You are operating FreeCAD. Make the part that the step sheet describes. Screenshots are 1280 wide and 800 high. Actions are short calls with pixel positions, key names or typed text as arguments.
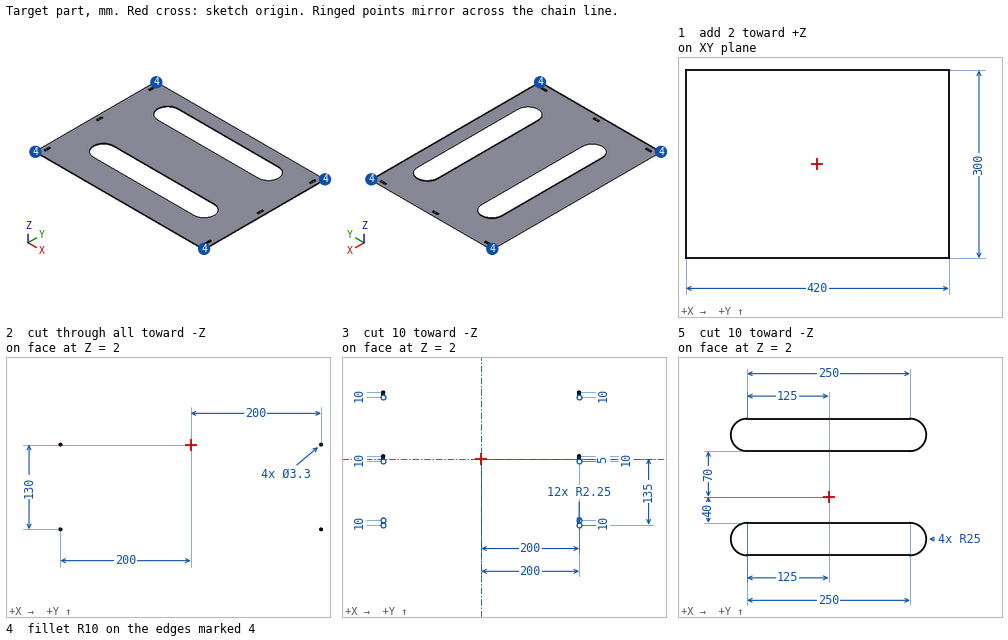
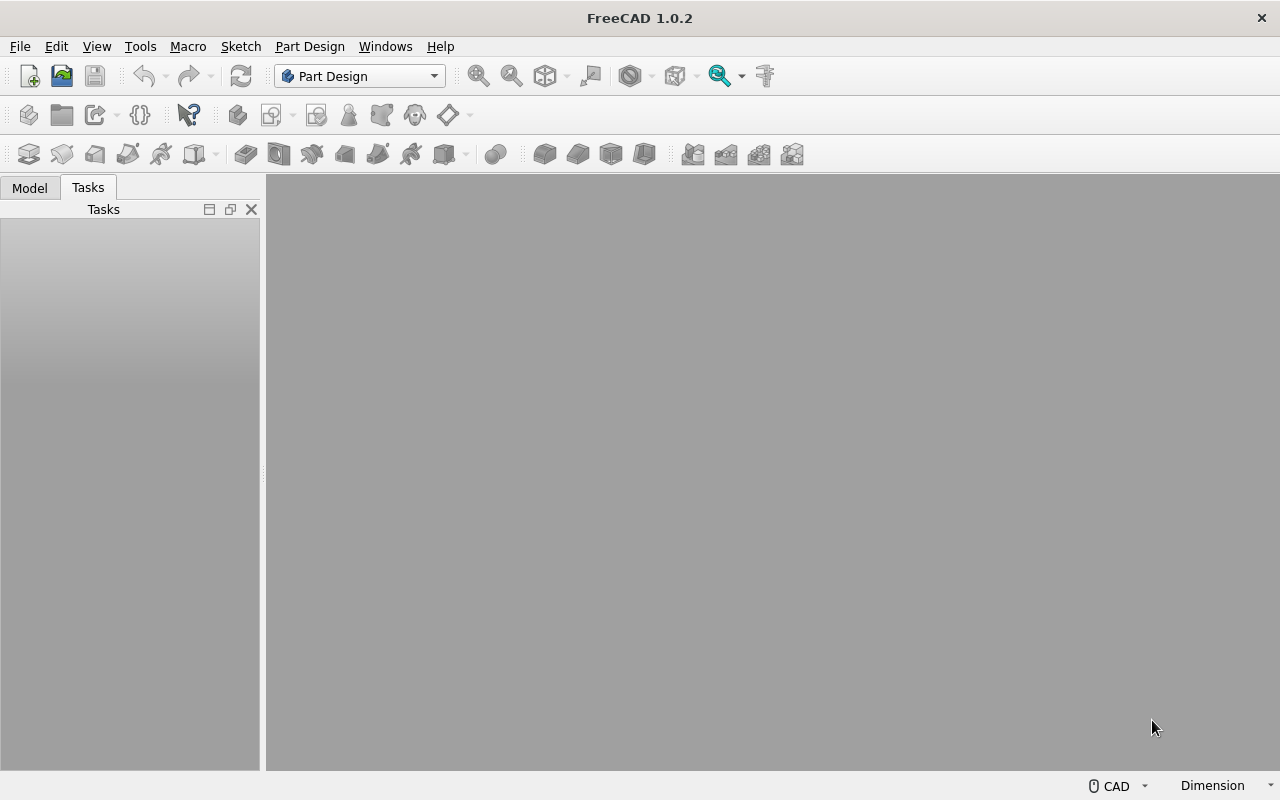
click(29, 76)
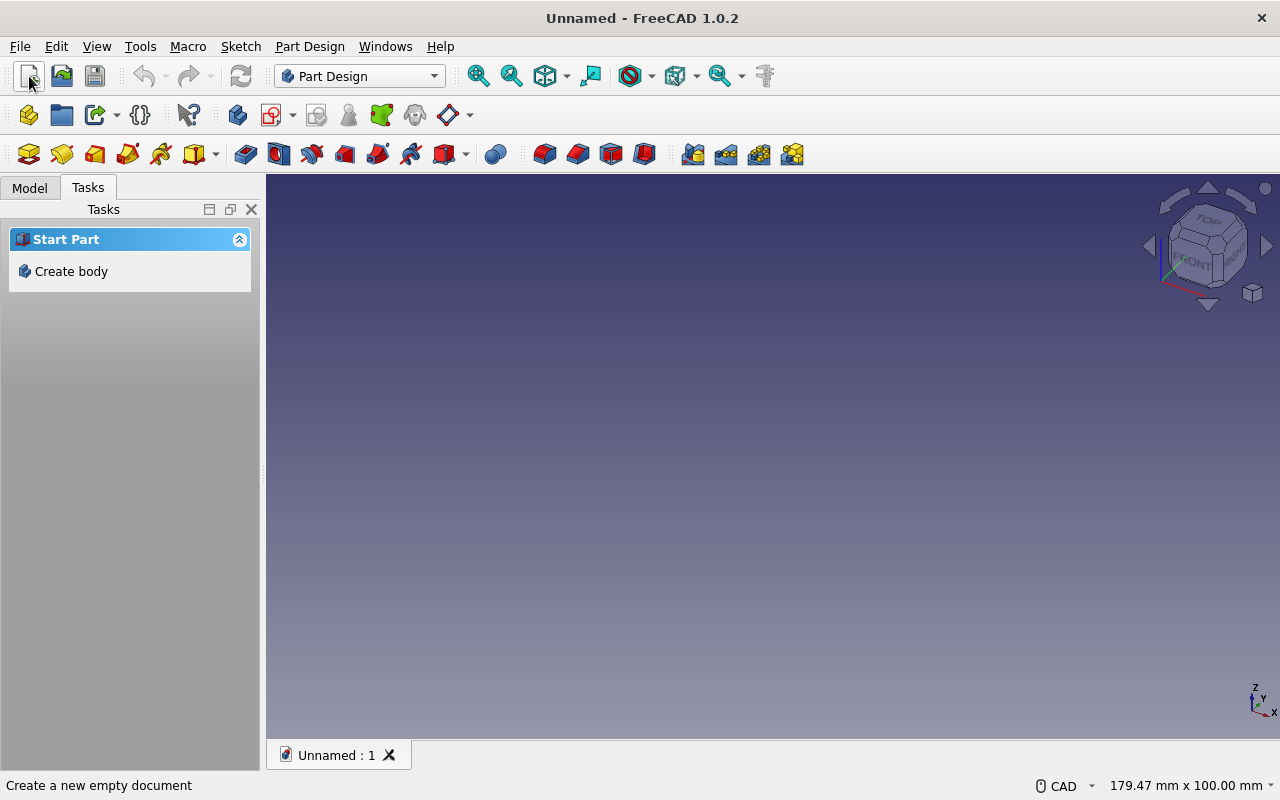
click(270, 116)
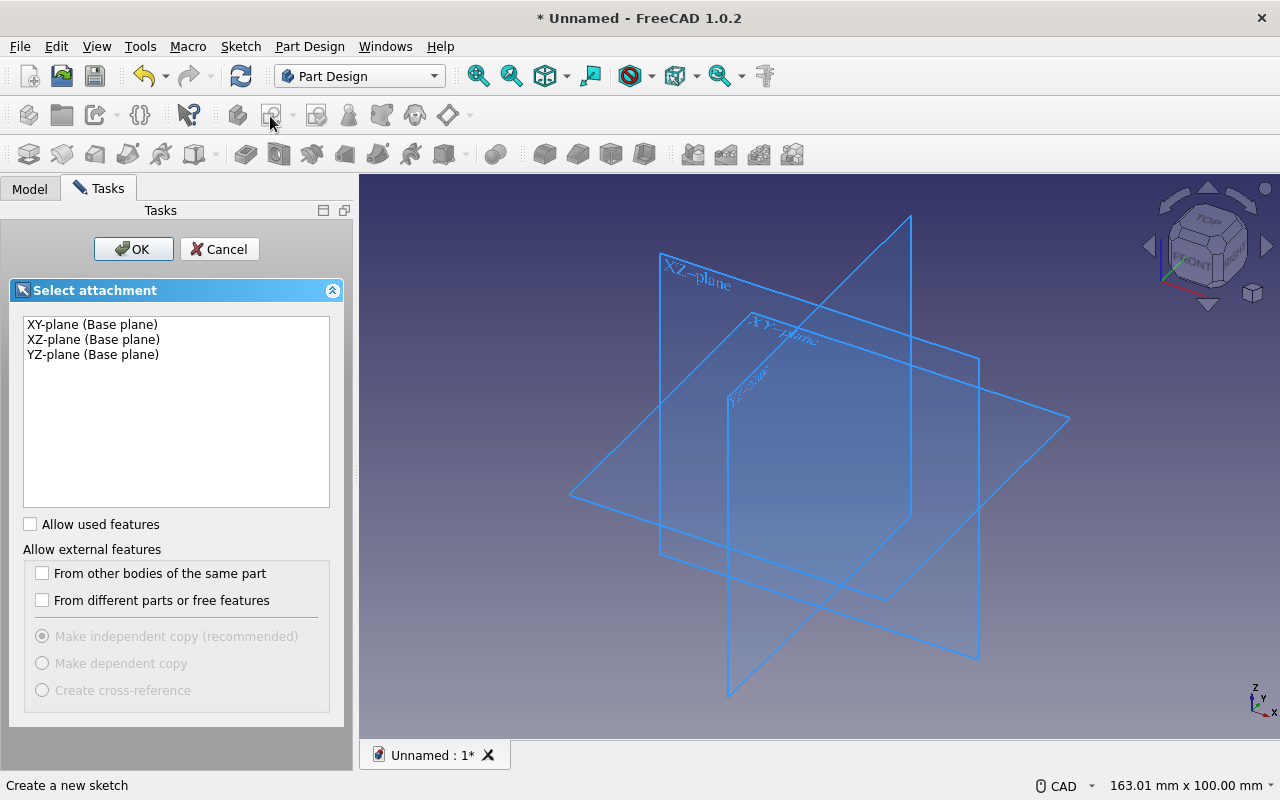
click(84, 324)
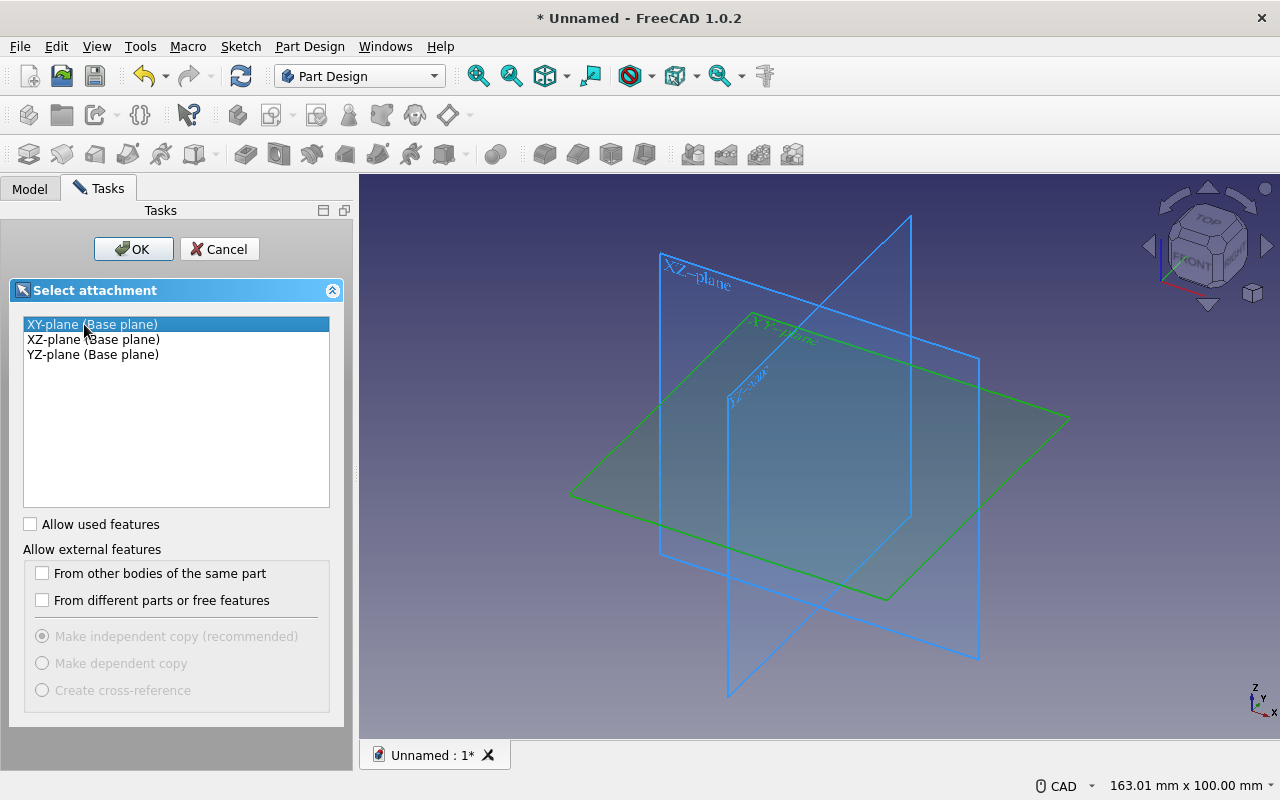
click(134, 249)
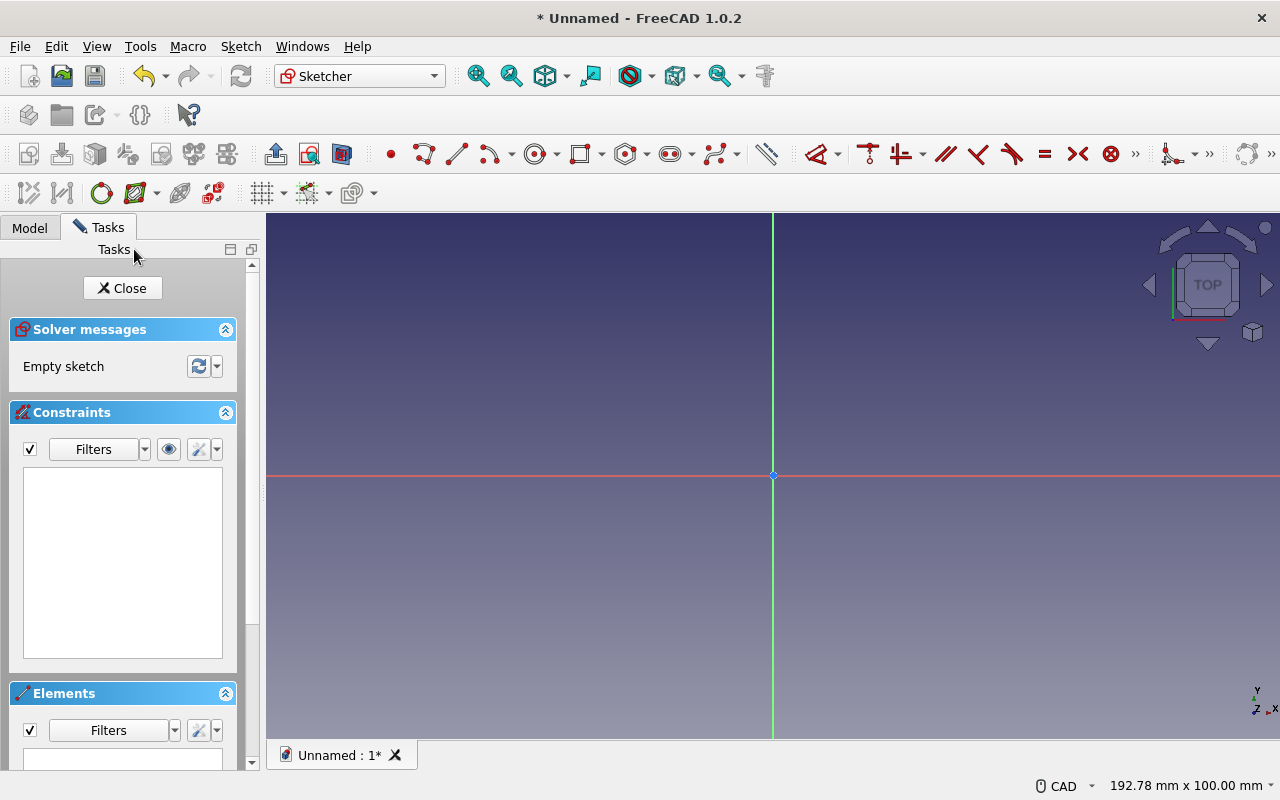
scroll(687, 476, down, 8)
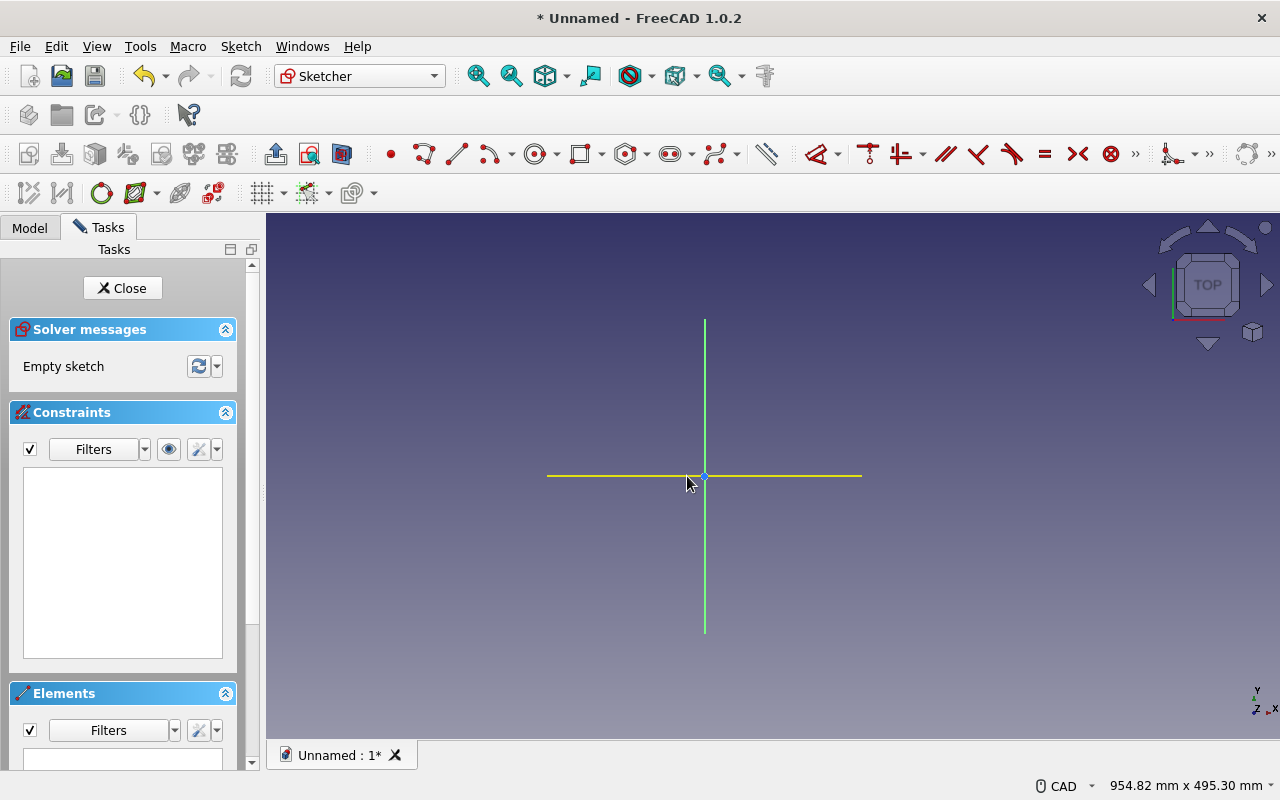
key(g)
key(v)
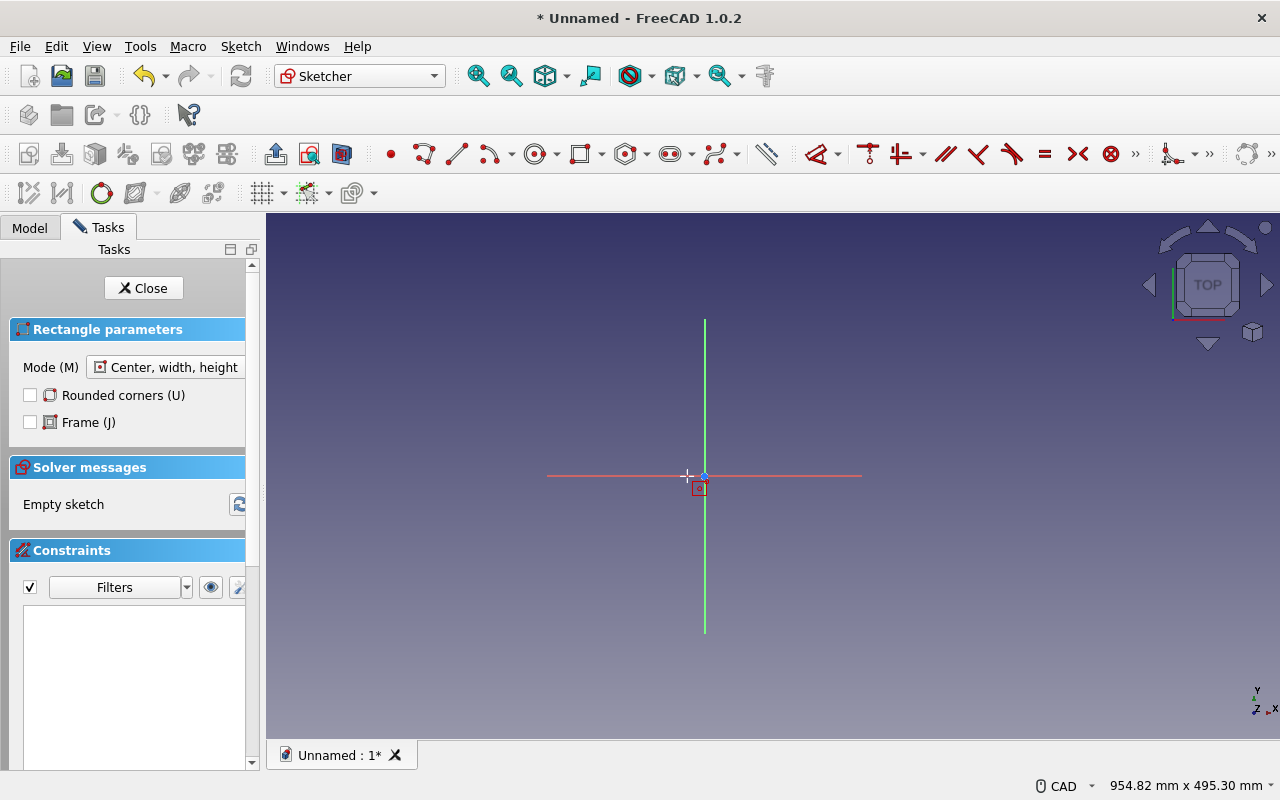
click(705, 476)
click(928, 317)
key(Escape)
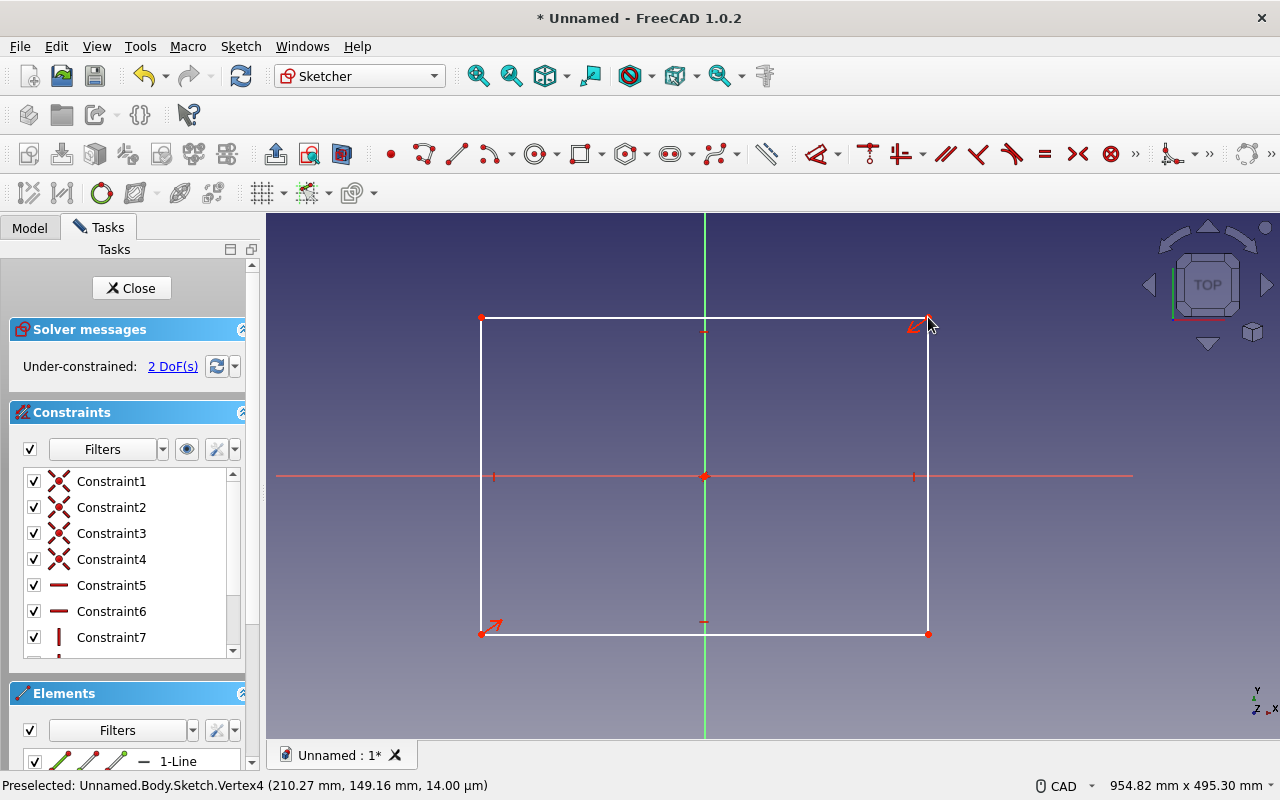
click(816, 154)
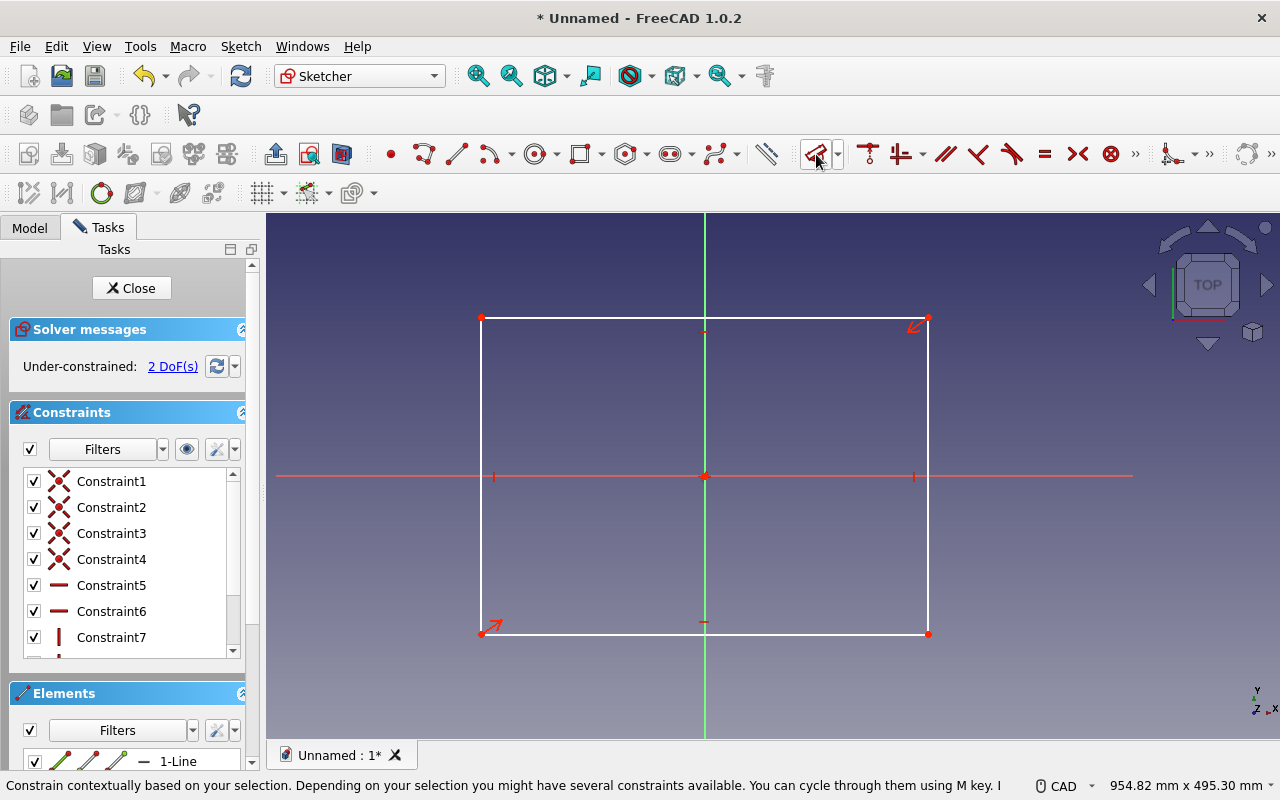
click(615, 635)
click(602, 669)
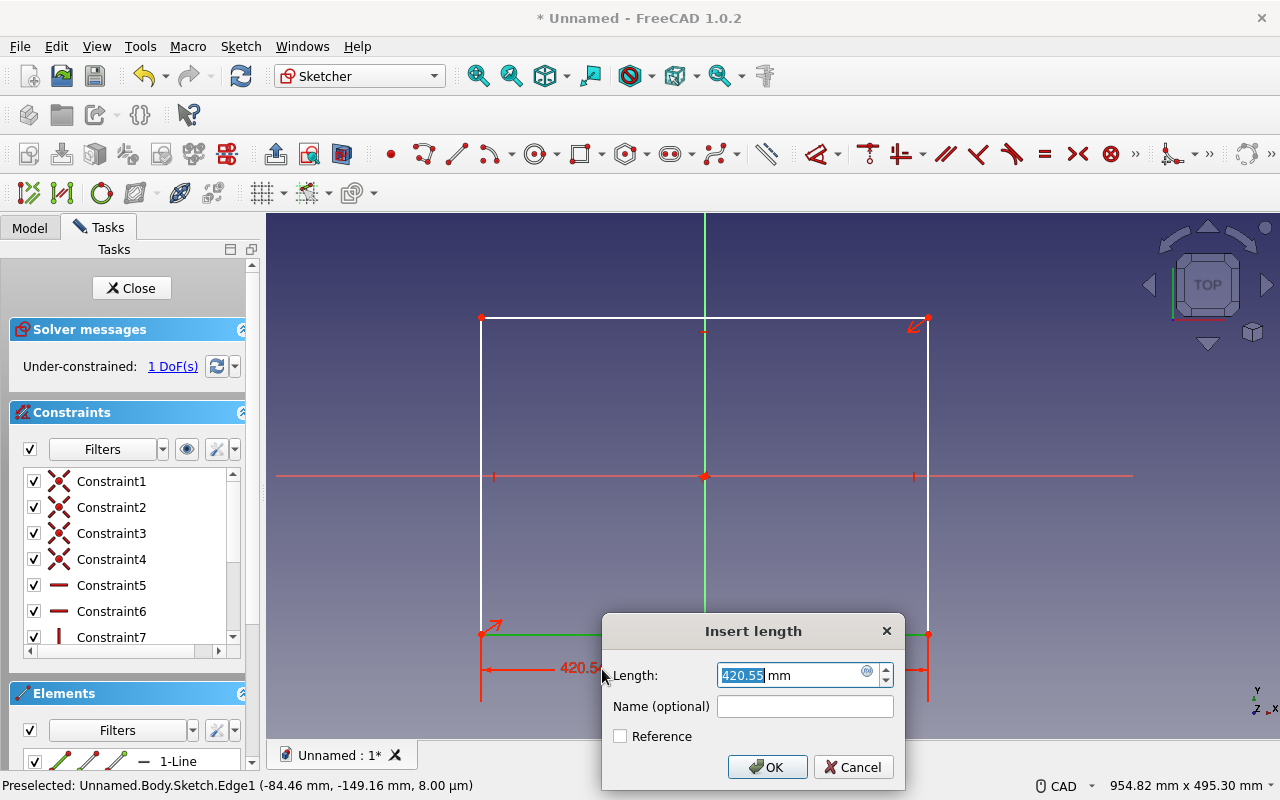
text(420)
key(Return)